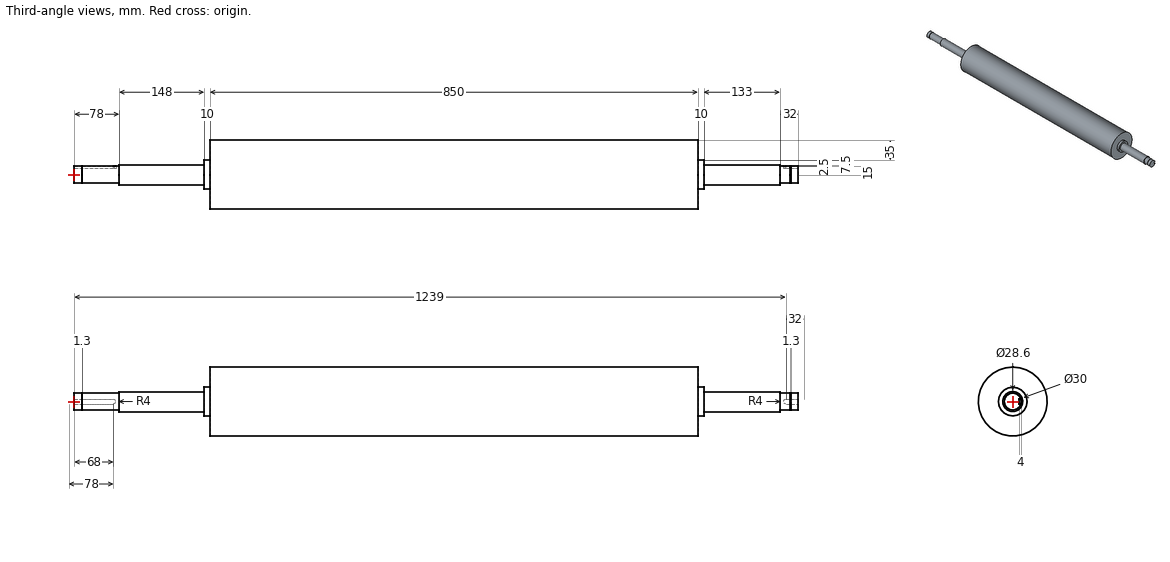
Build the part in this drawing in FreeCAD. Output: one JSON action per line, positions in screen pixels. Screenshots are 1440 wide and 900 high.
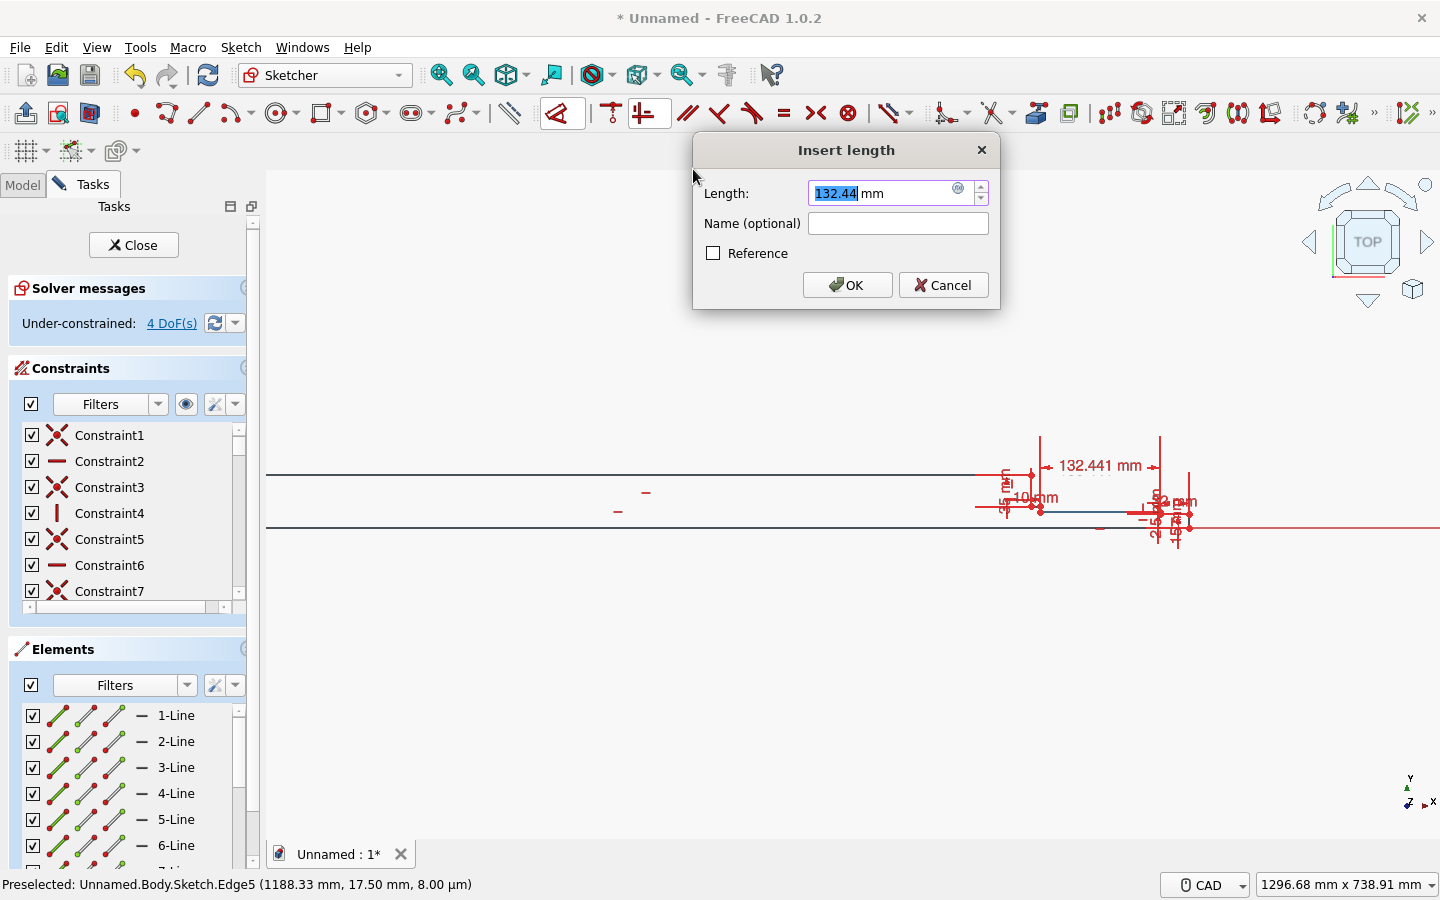
{"action": "type", "text": "133"}
{"action": "key", "text": "Return"}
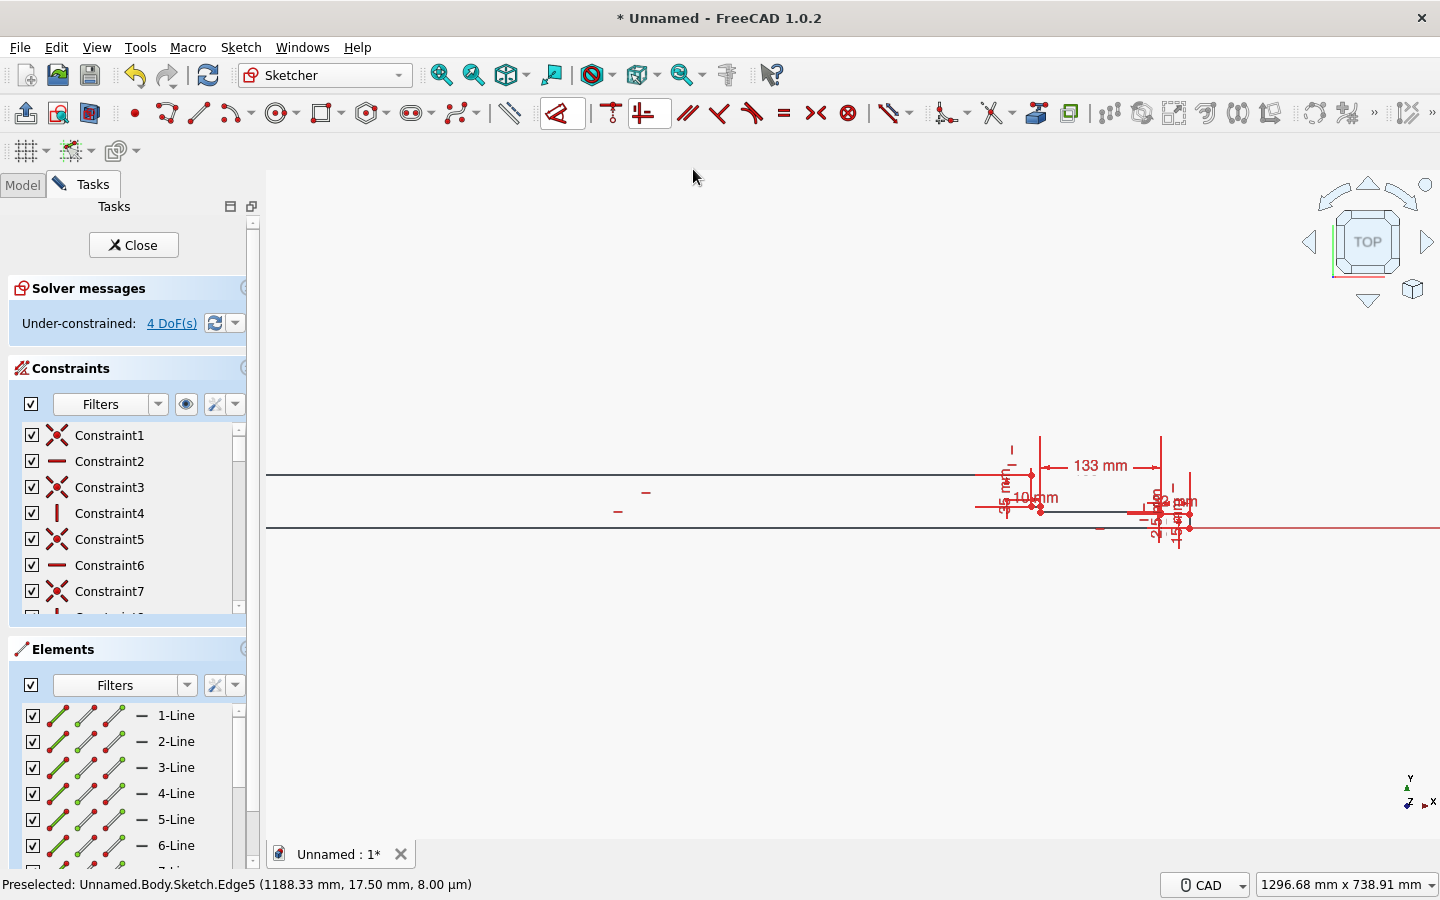
{"action": "scroll", "coordinate": [1040, 510], "scroll_direction": "up", "scroll_amount": 9}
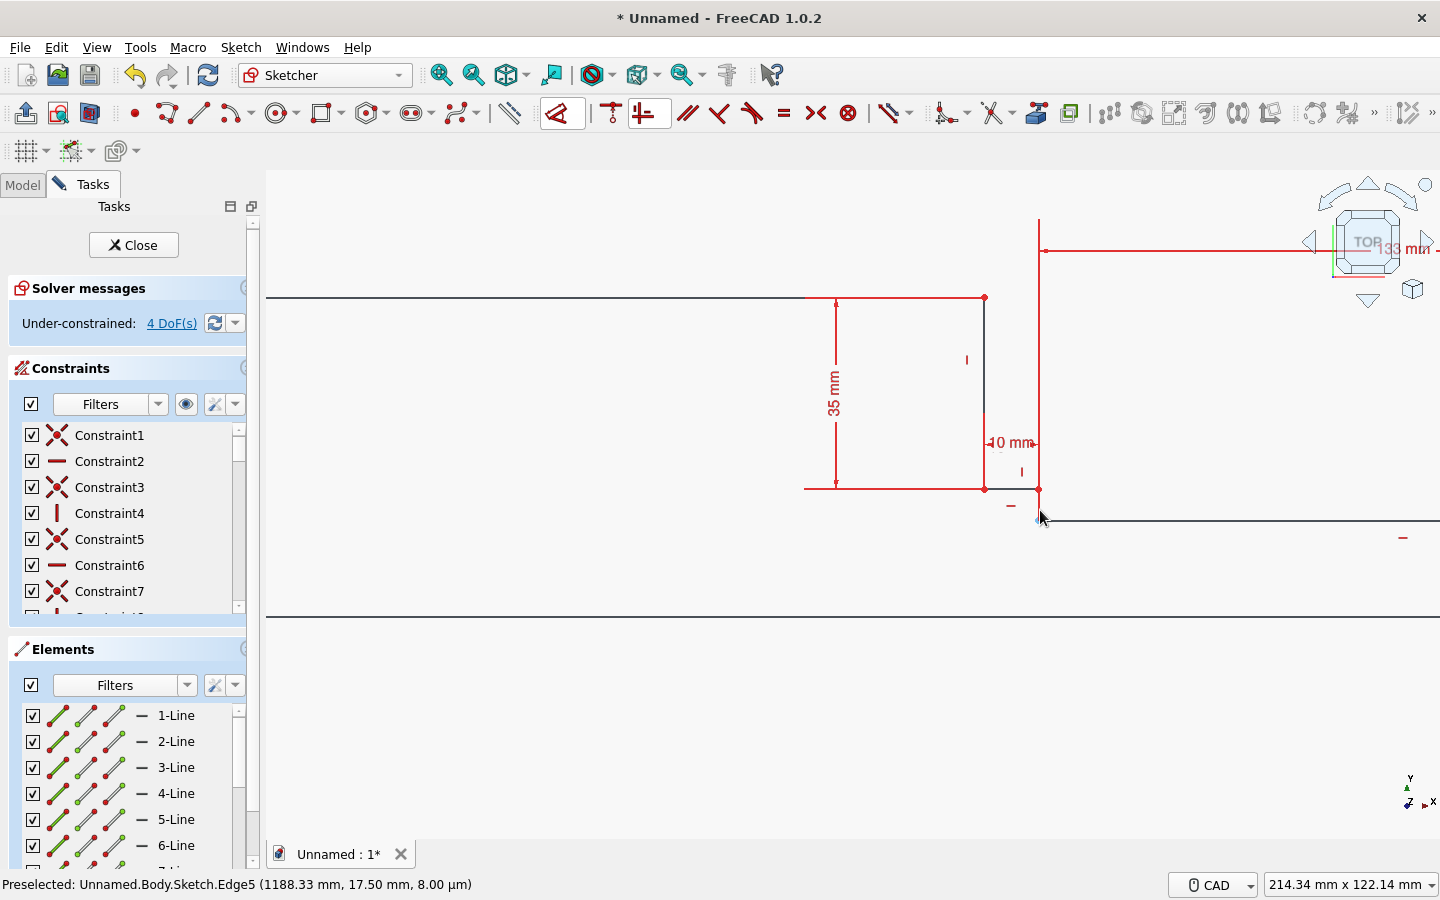
{"action": "left_click", "coordinate": [1039, 505]}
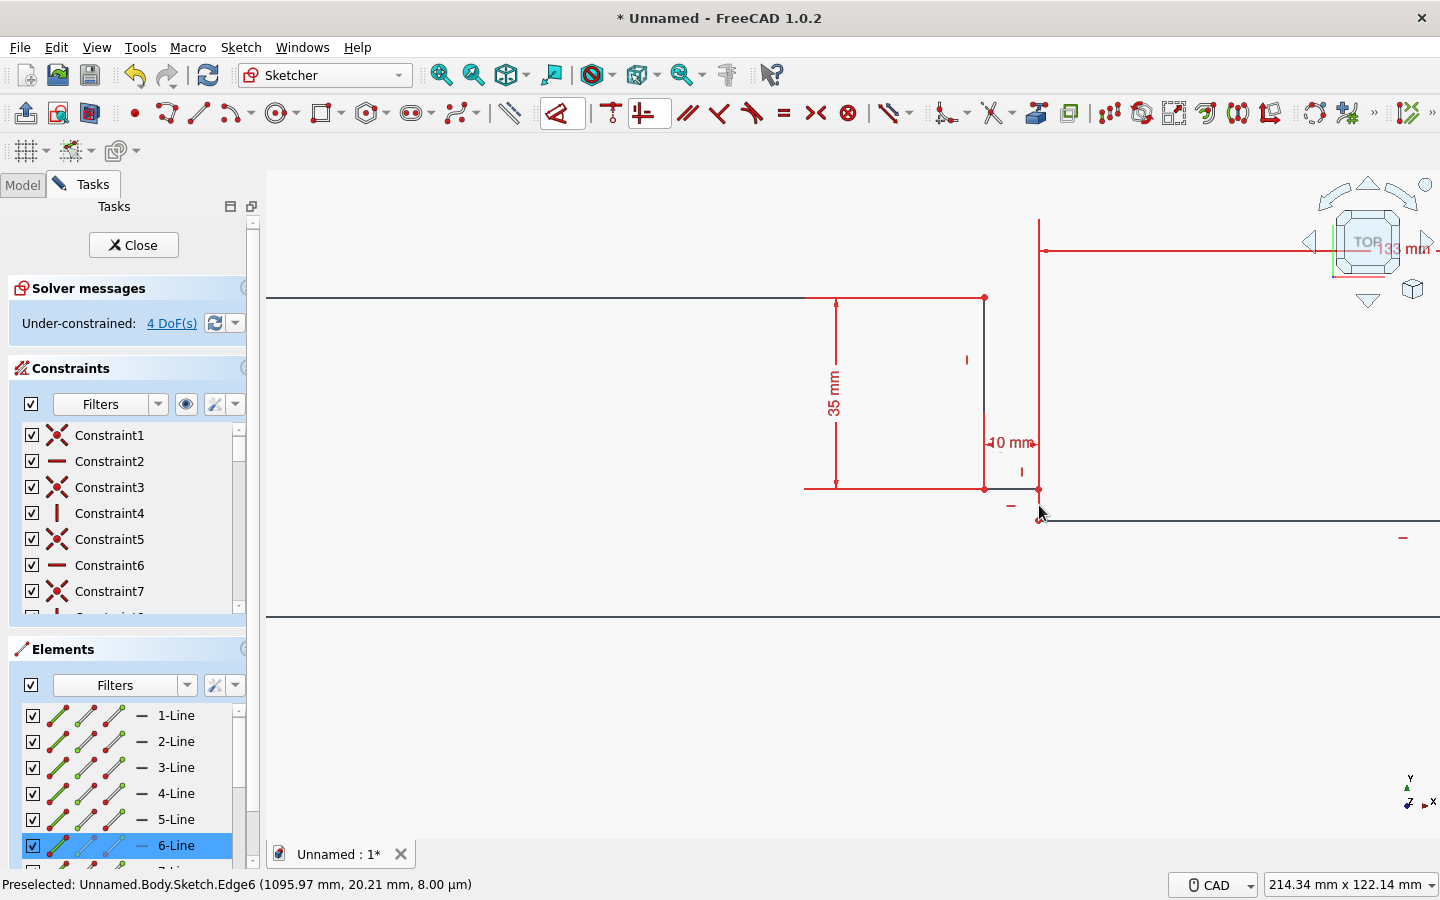
{"action": "key", "text": "i"}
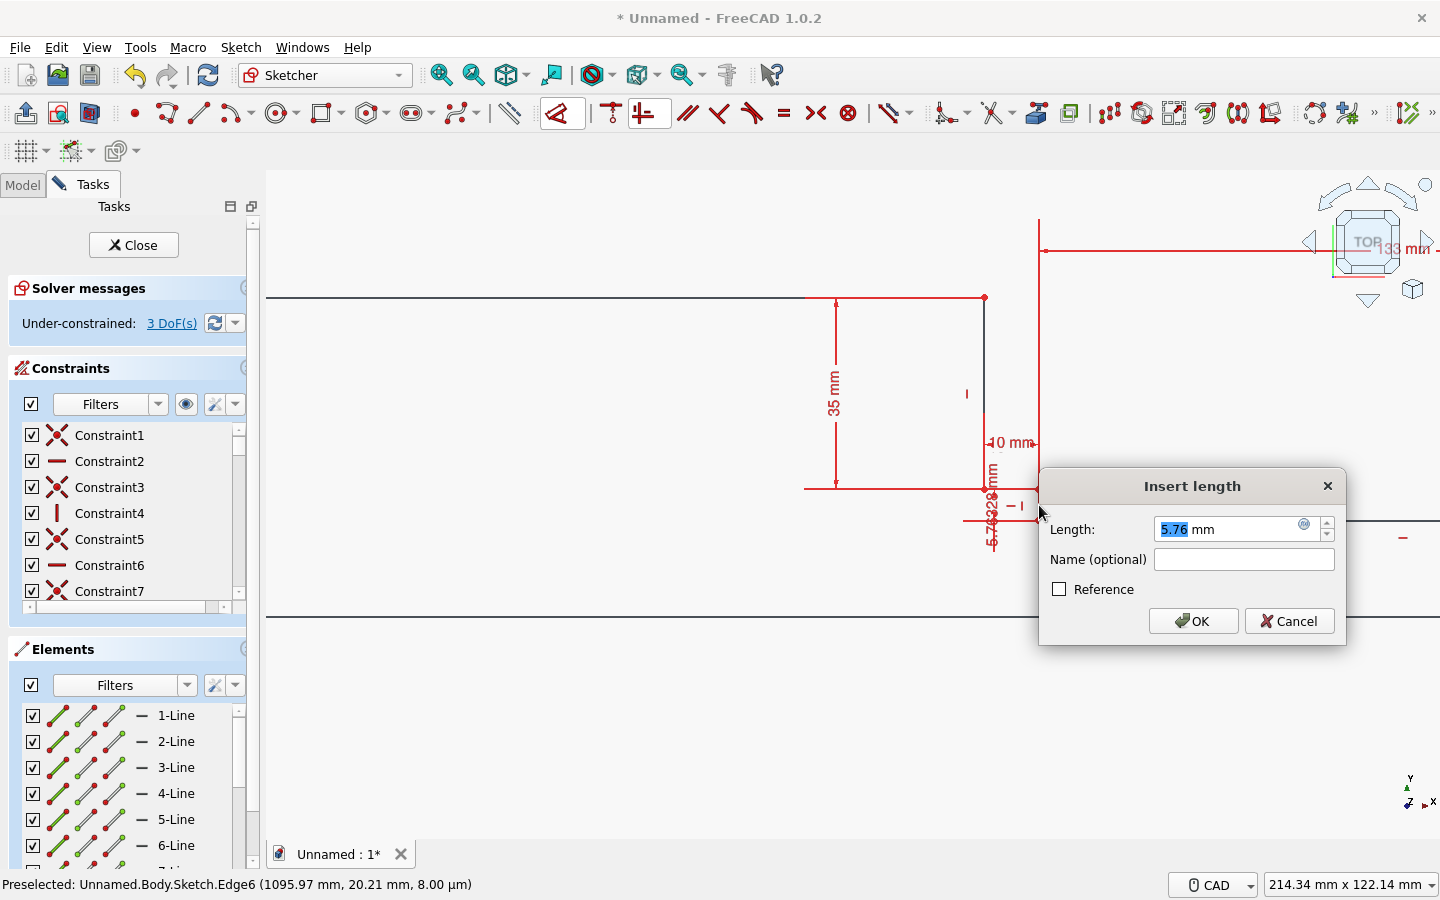
{"action": "type", "text": "7.5"}
{"action": "key", "text": "Return"}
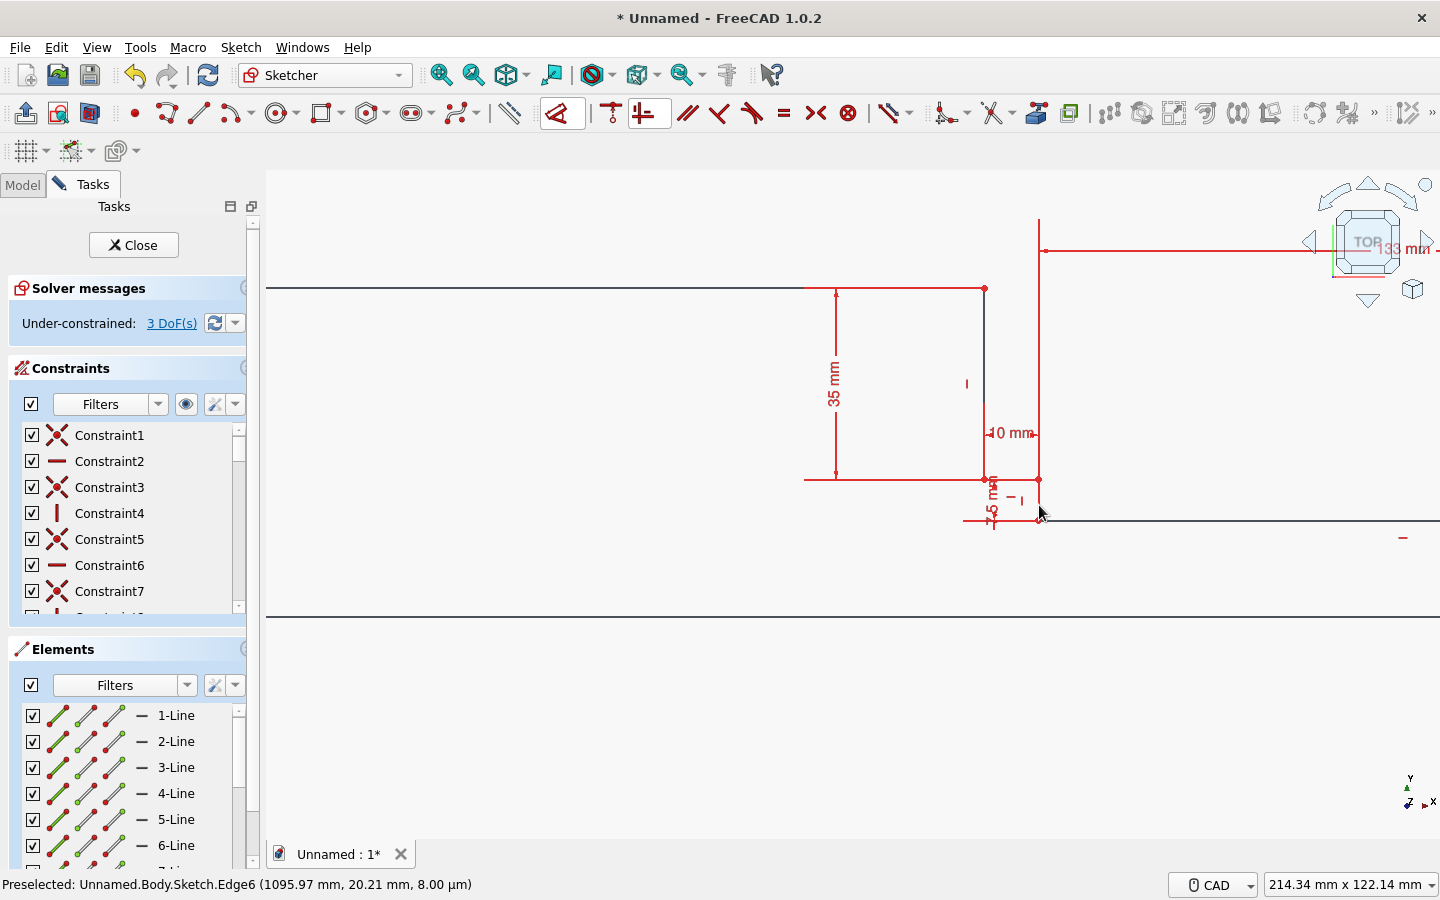
{"action": "scroll", "coordinate": [1013, 510], "scroll_direction": "down", "scroll_amount": 12}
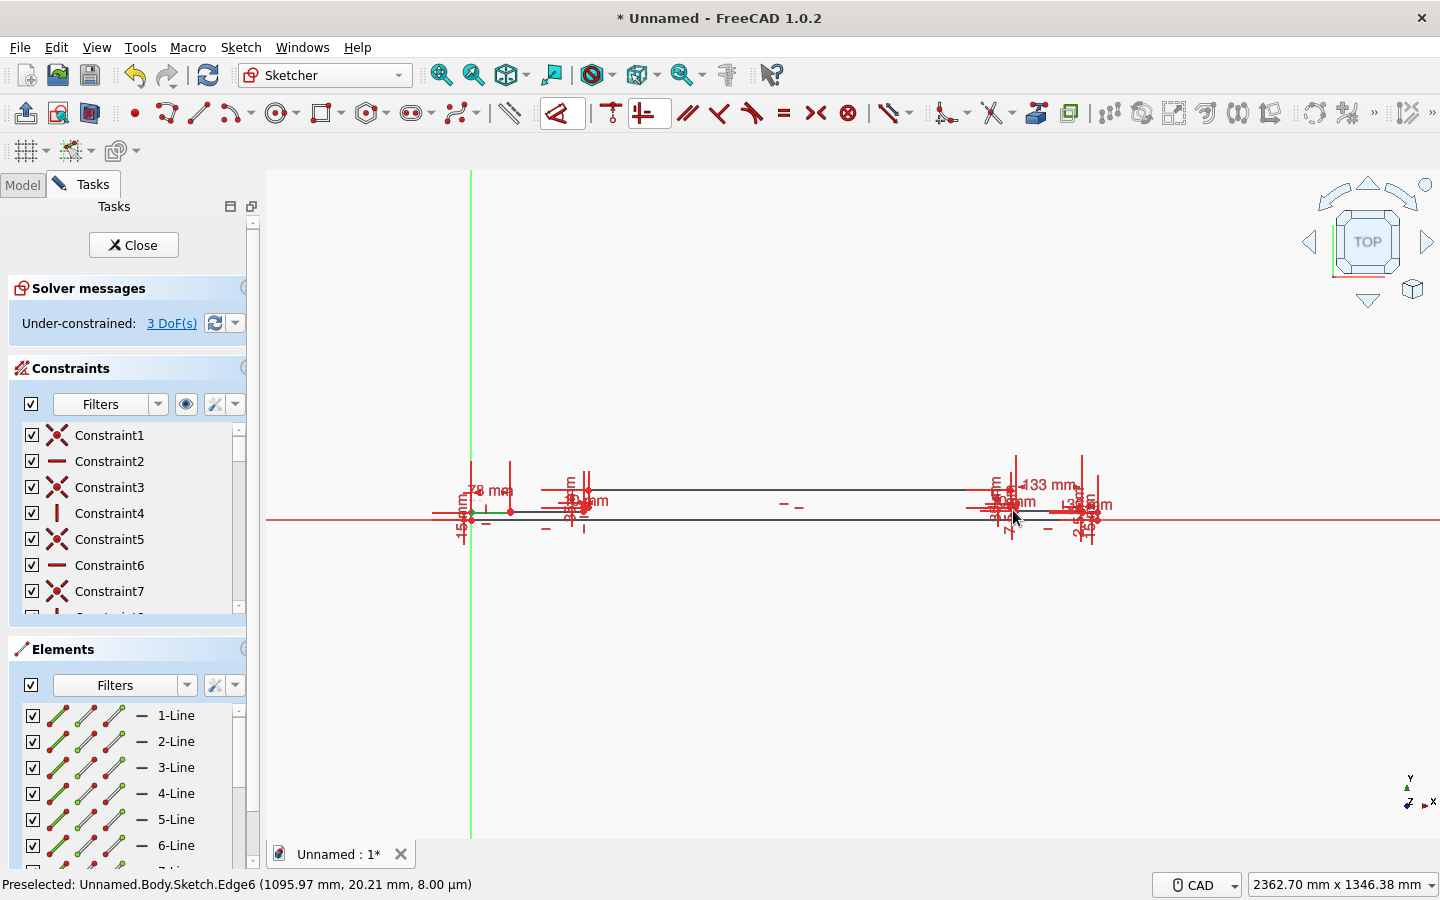
{"action": "left_click", "coordinate": [884, 490]}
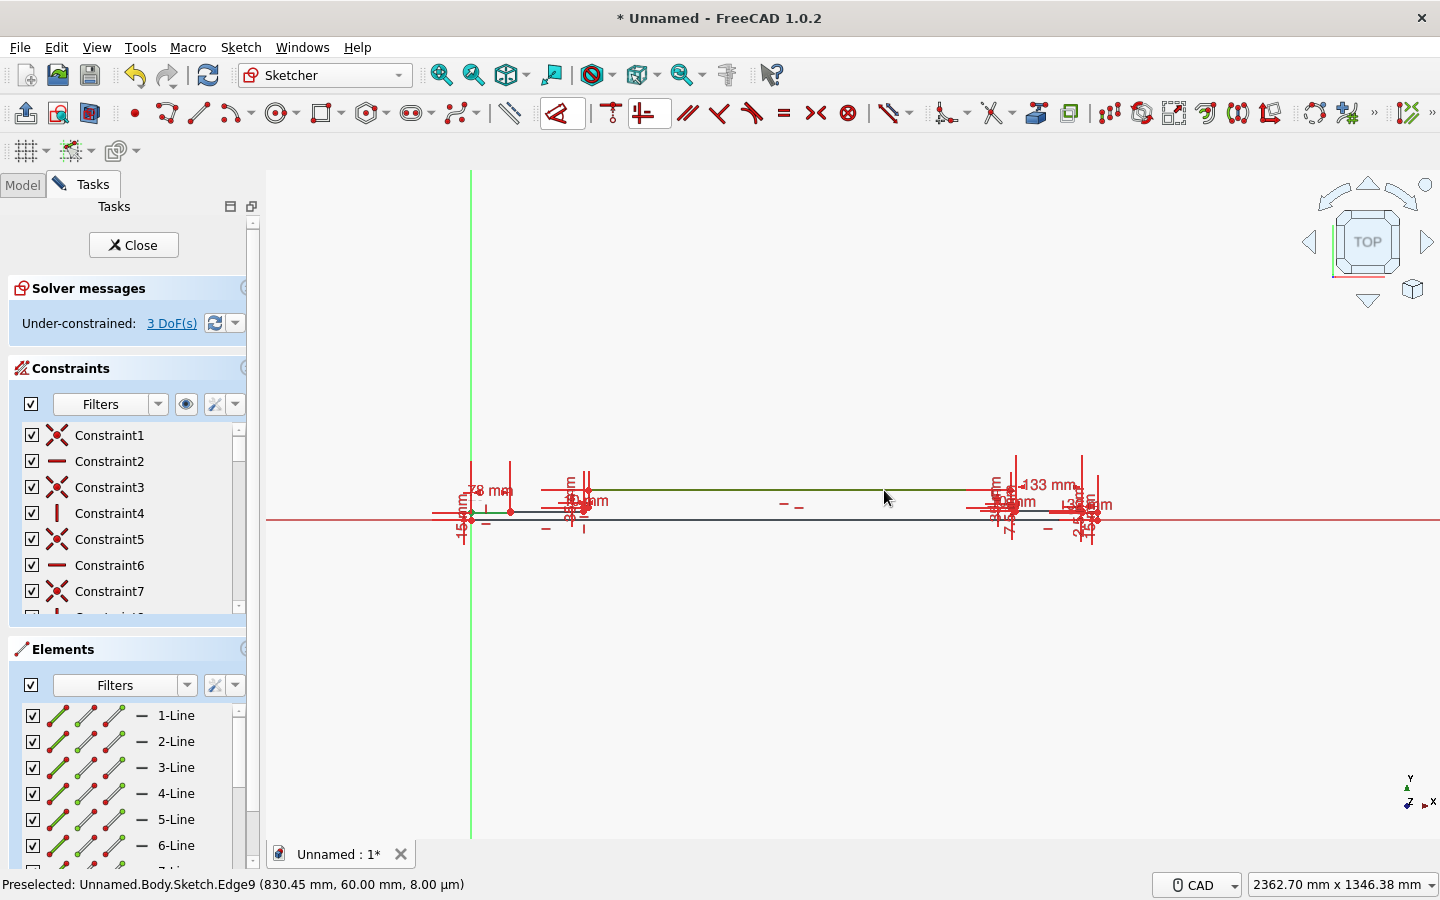
{"action": "key", "text": "l"}